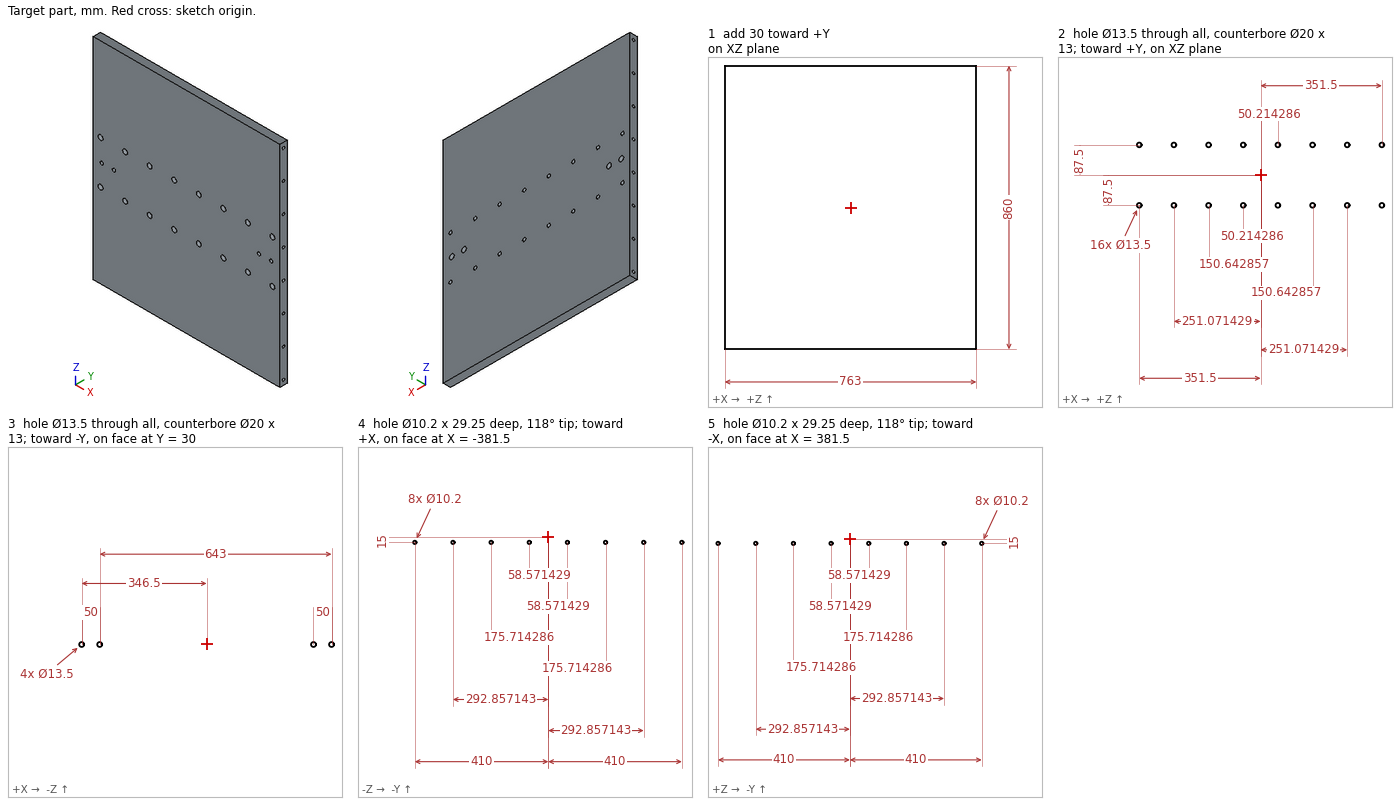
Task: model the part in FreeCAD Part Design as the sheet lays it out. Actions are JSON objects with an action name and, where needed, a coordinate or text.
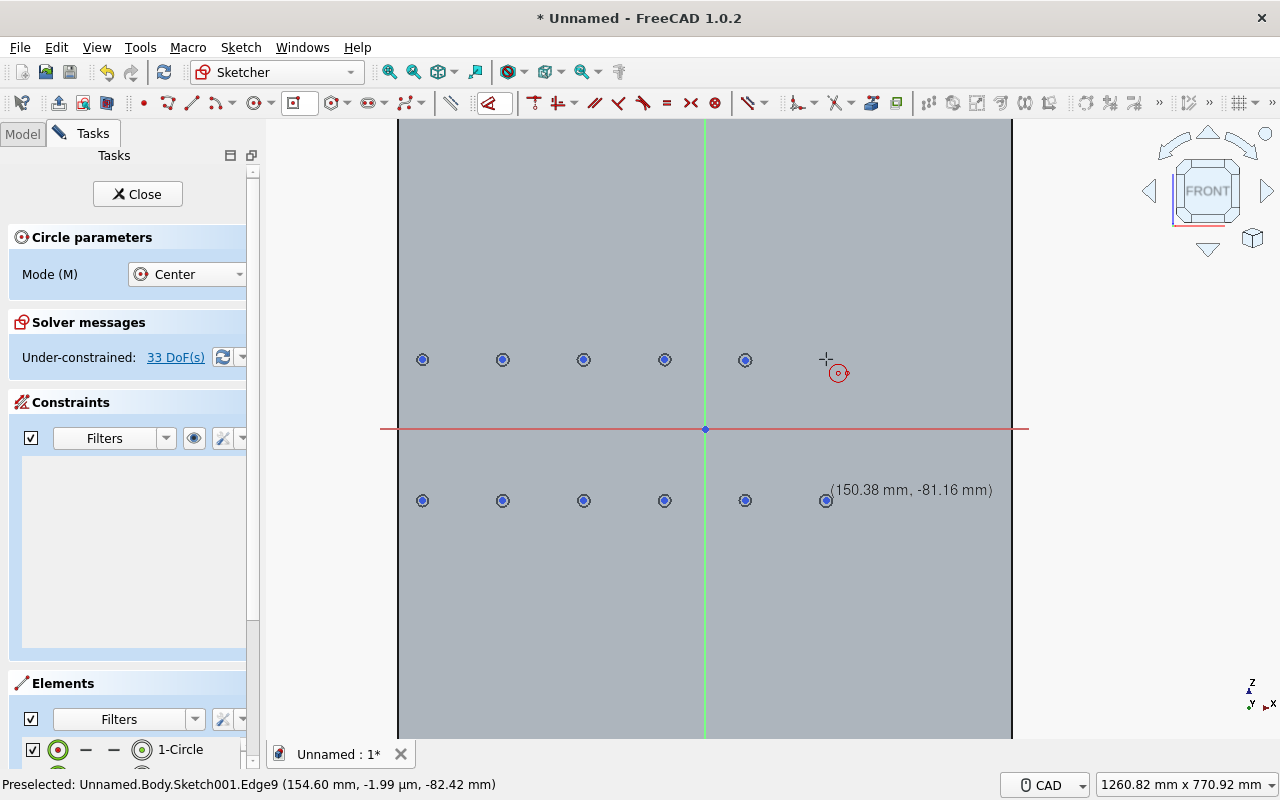
{"action": "left_click", "coordinate": [826, 359]}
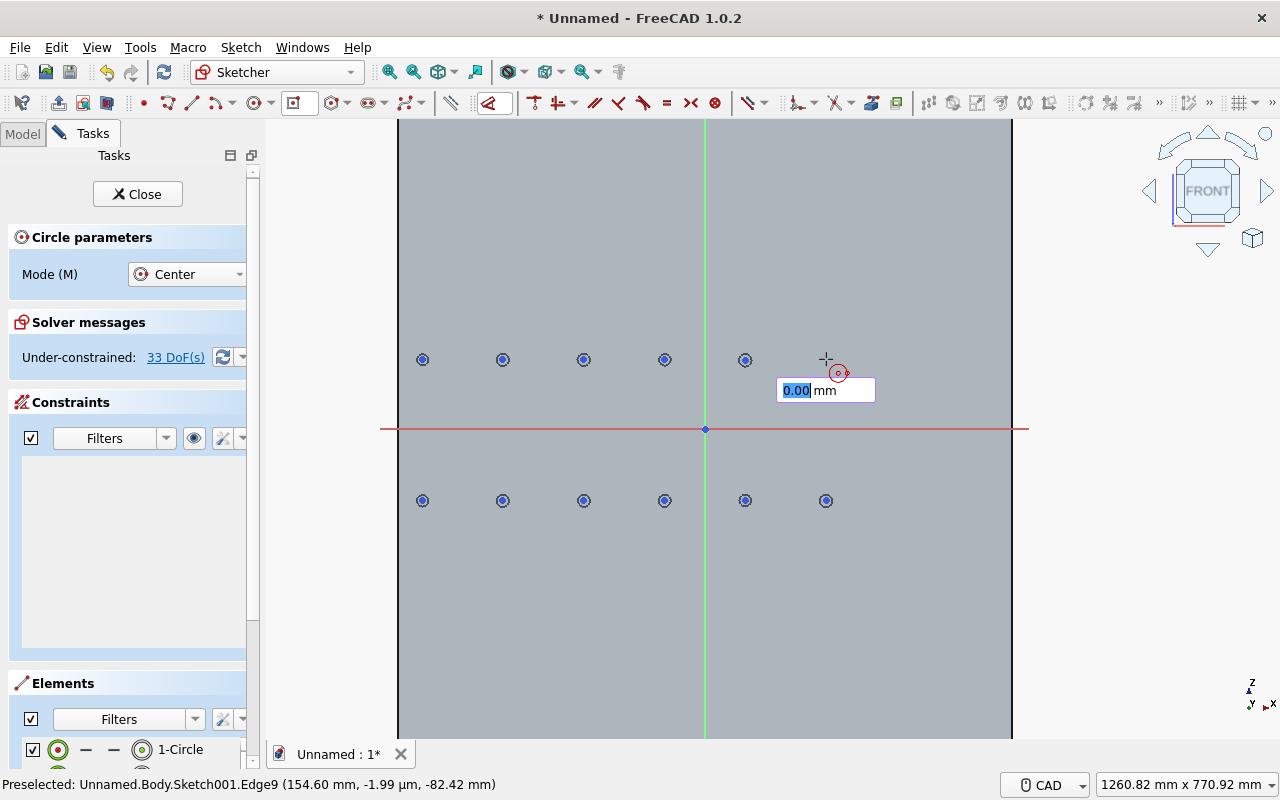
{"action": "scroll", "coordinate": [830, 355], "scroll_direction": "up", "scroll_amount": 6}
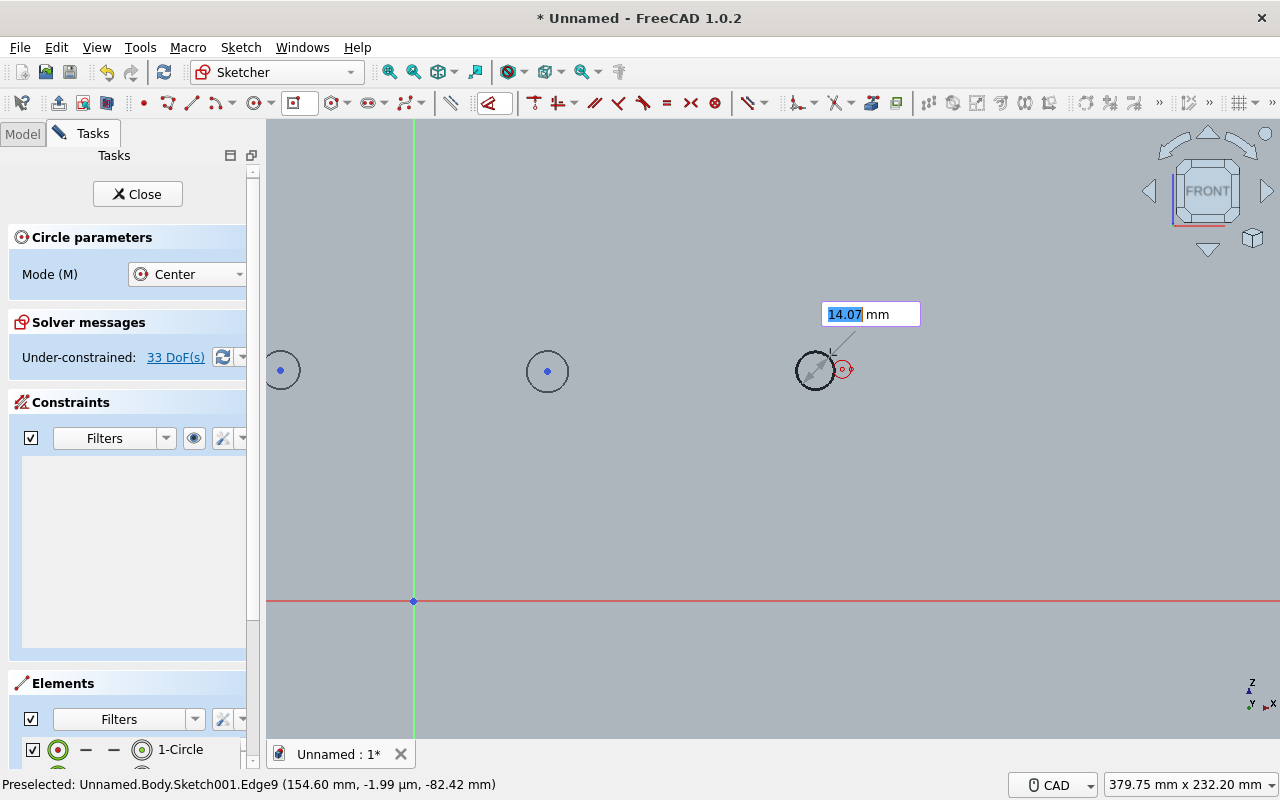
{"action": "left_click", "coordinate": [829, 355]}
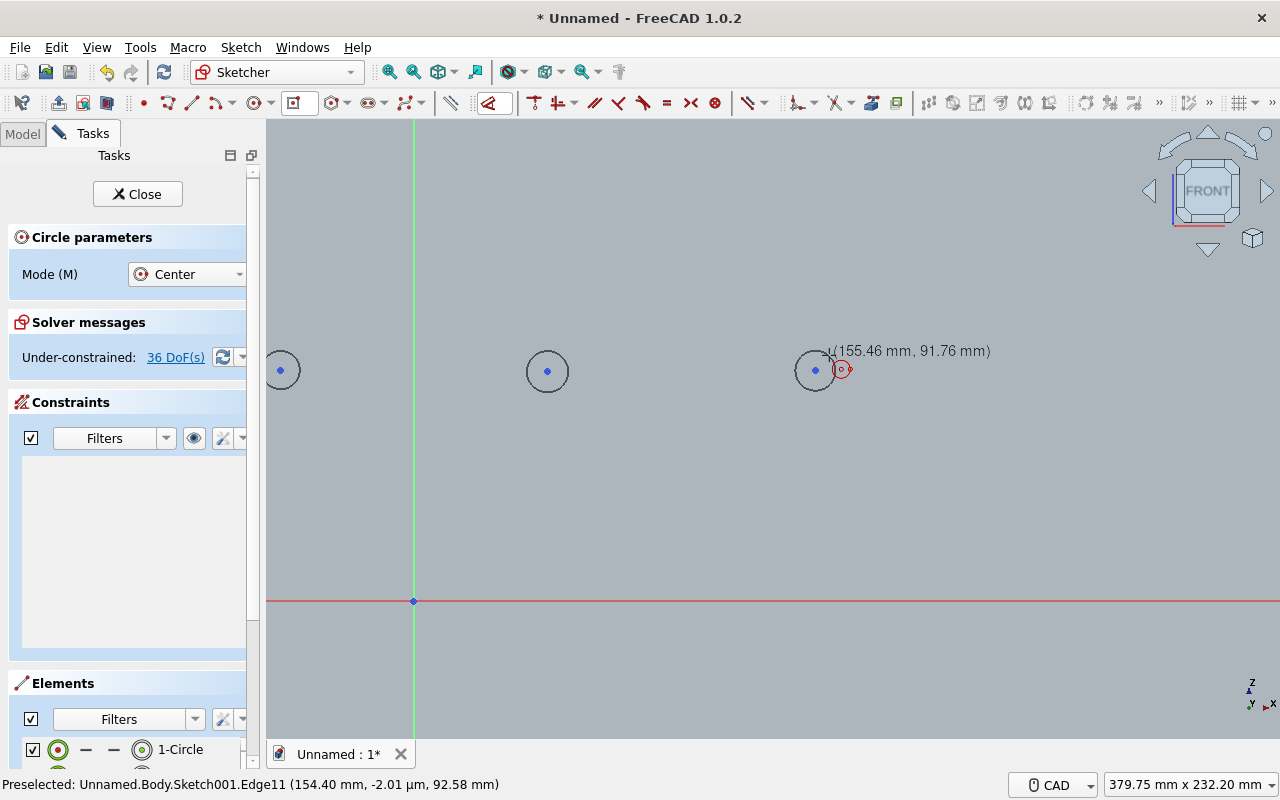
{"action": "scroll", "coordinate": [830, 355], "scroll_direction": "down", "scroll_amount": 6}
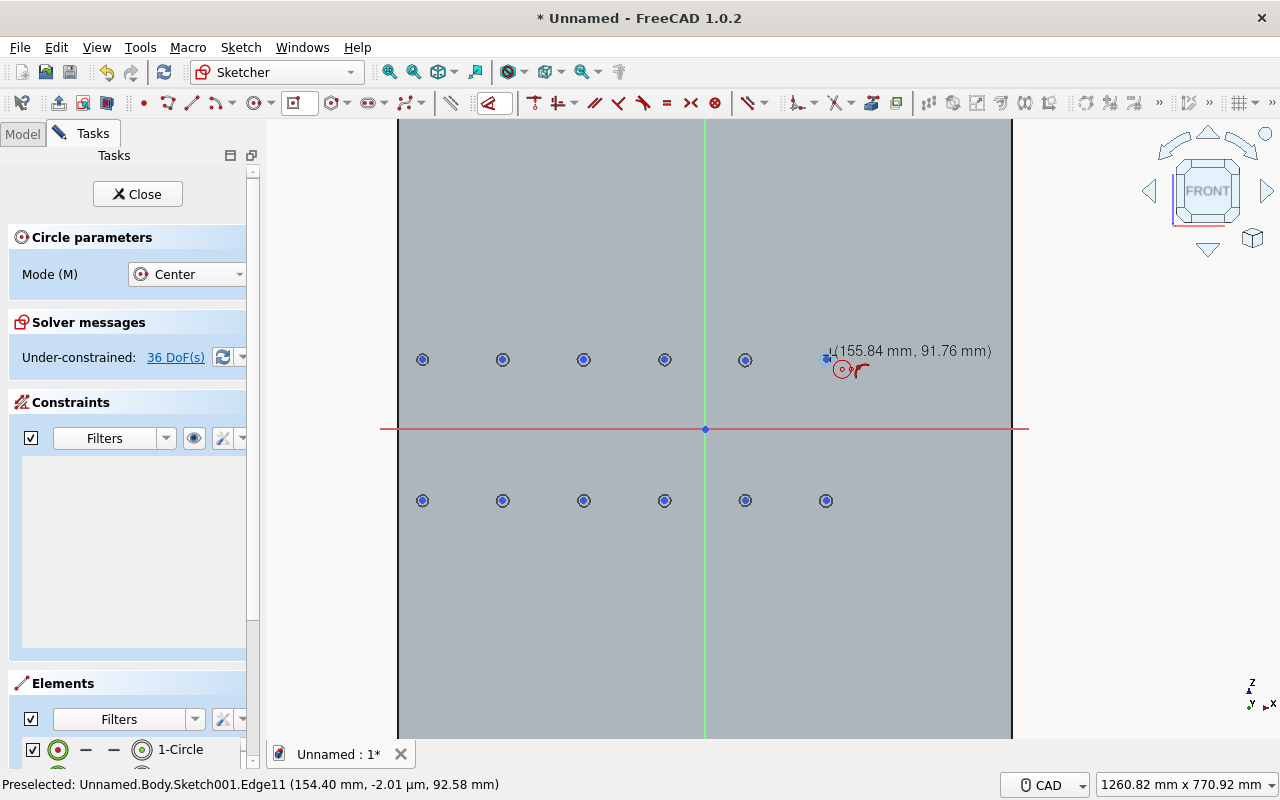
{"action": "scroll", "coordinate": [907, 500], "scroll_direction": "up", "scroll_amount": 8}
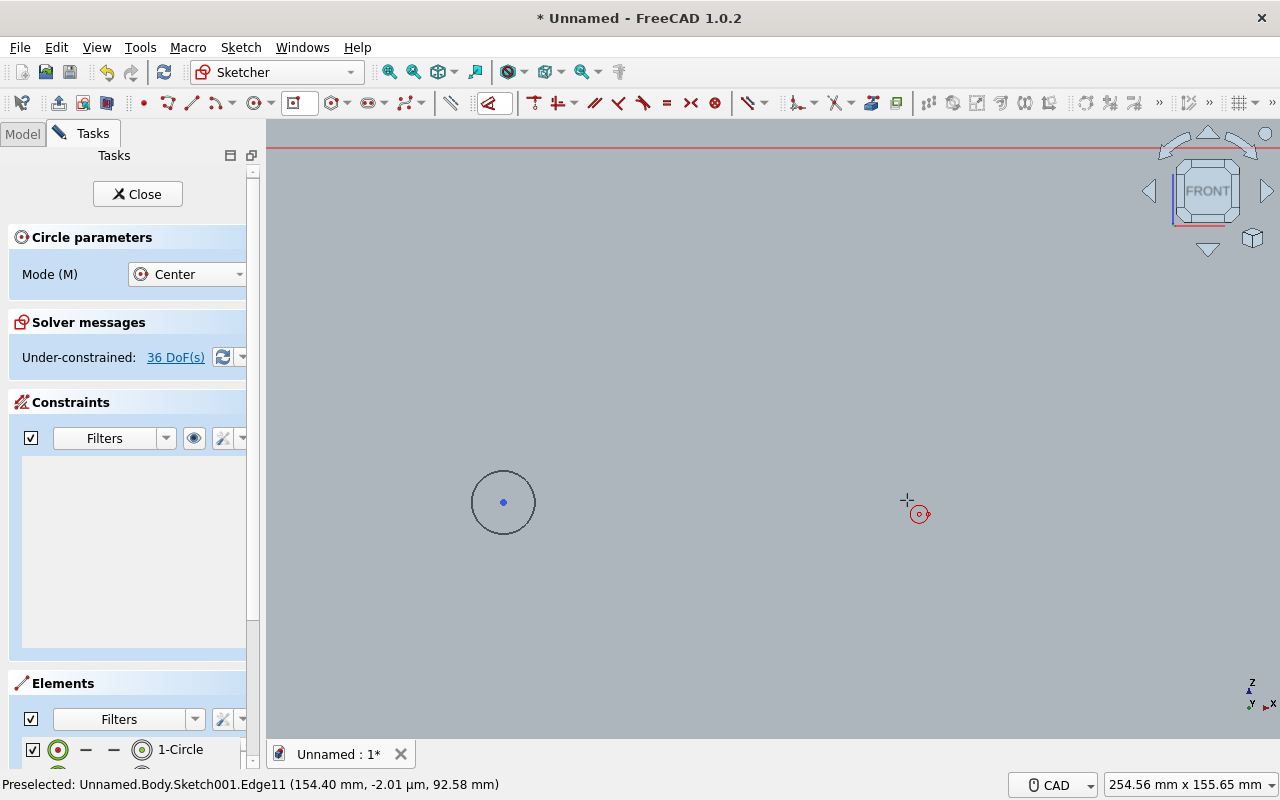
{"action": "scroll", "coordinate": [907, 500], "scroll_direction": "down", "scroll_amount": 8}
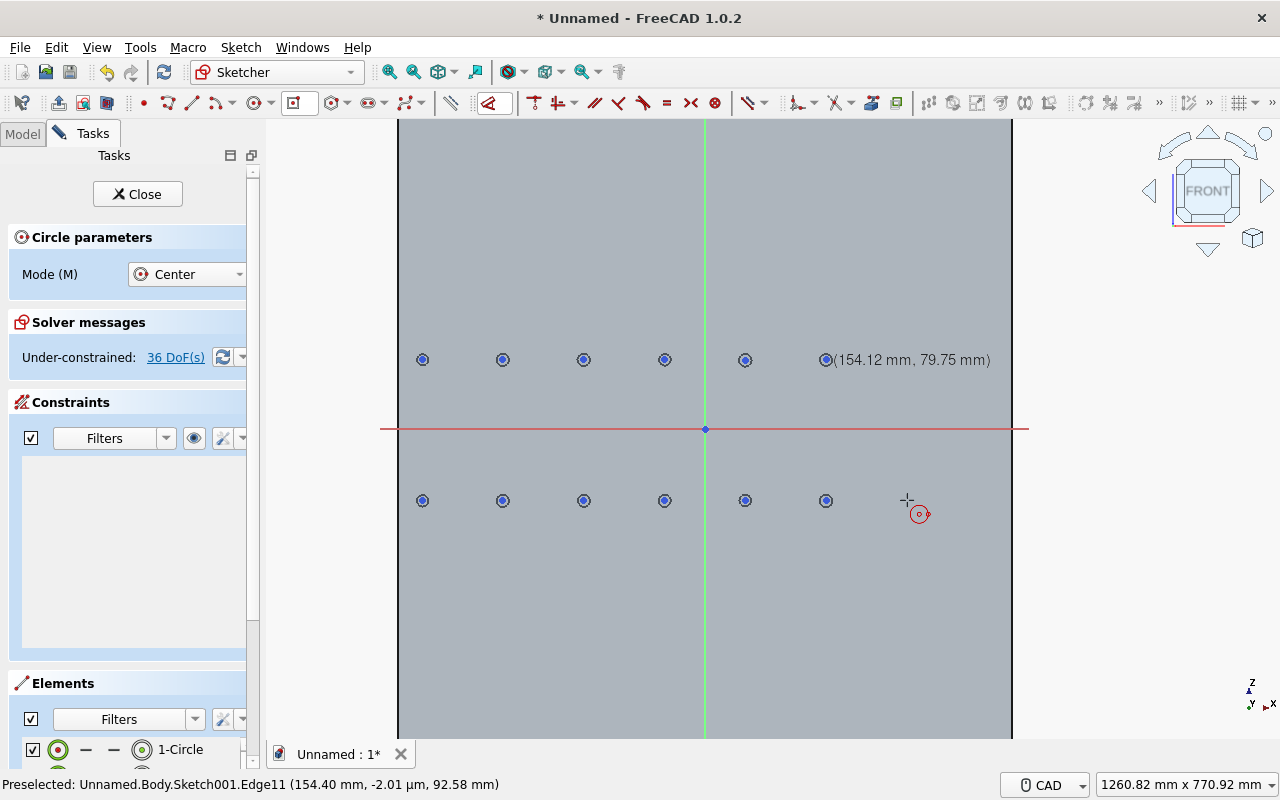
{"action": "left_click", "coordinate": [907, 500]}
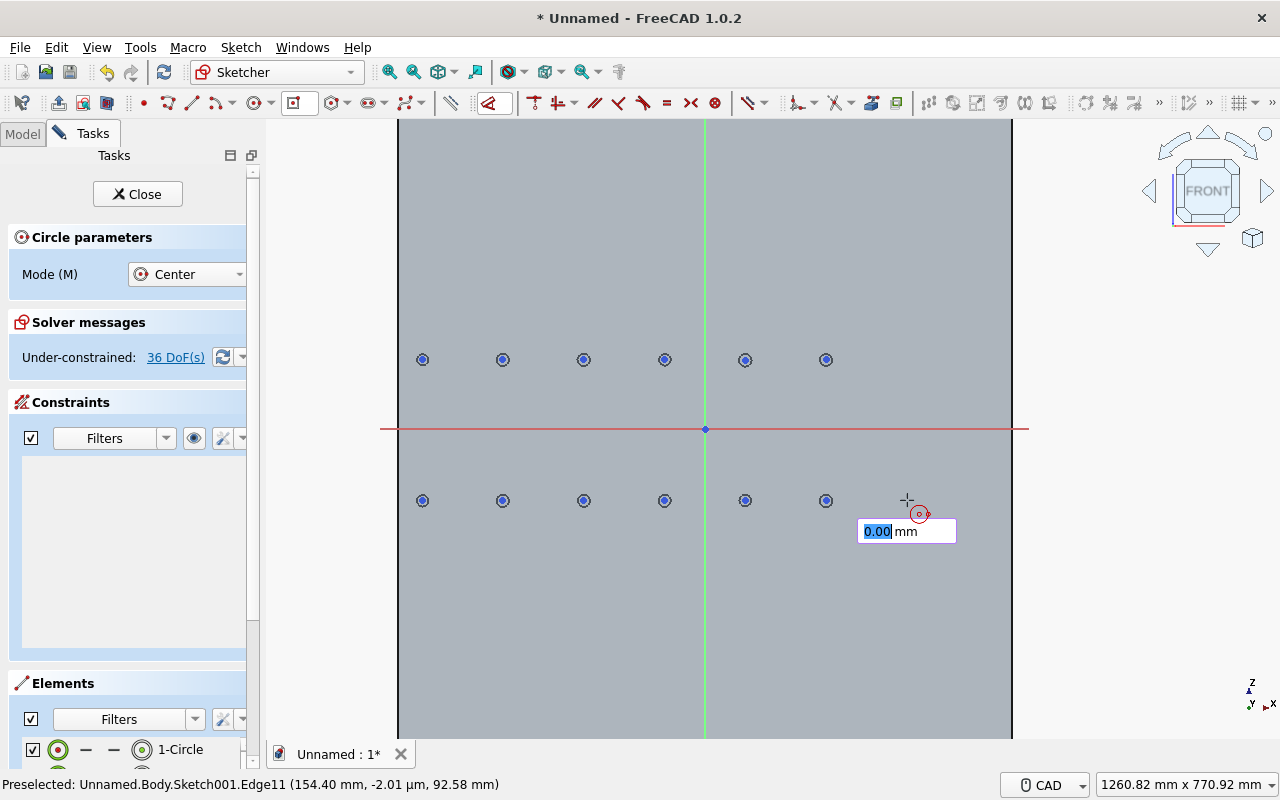
{"action": "scroll", "coordinate": [911, 496], "scroll_direction": "up", "scroll_amount": 6}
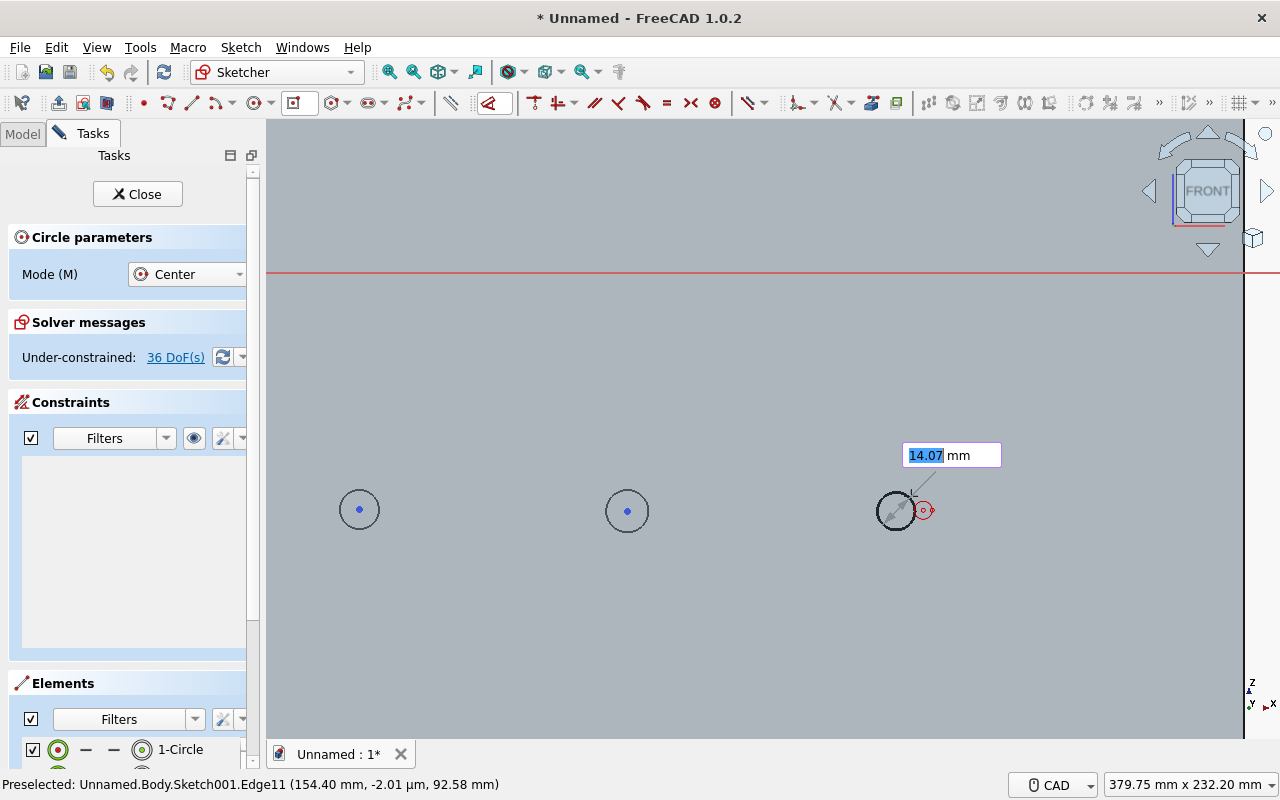
{"action": "left_click", "coordinate": [909, 494]}